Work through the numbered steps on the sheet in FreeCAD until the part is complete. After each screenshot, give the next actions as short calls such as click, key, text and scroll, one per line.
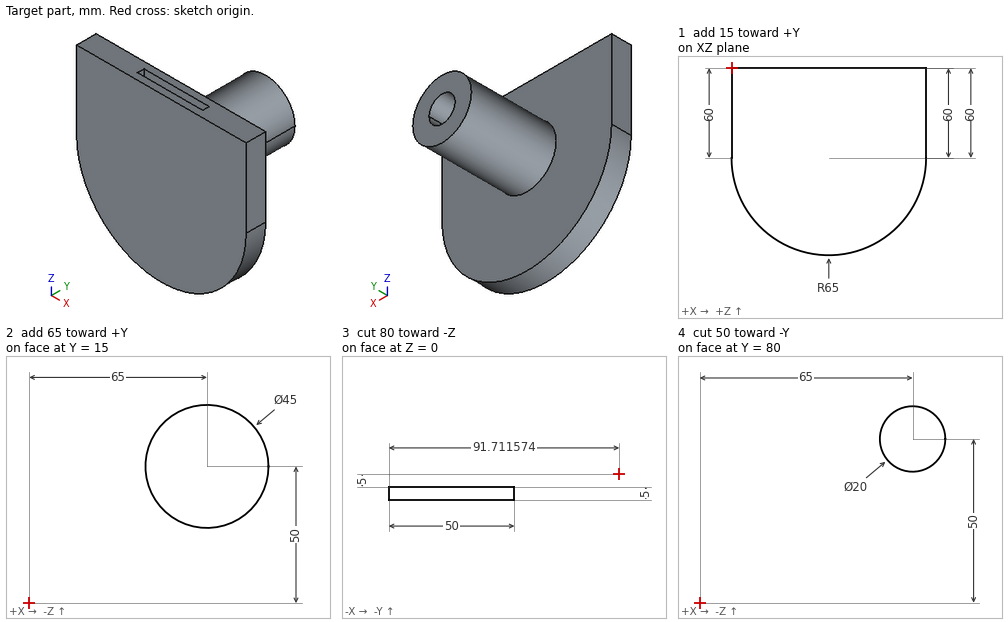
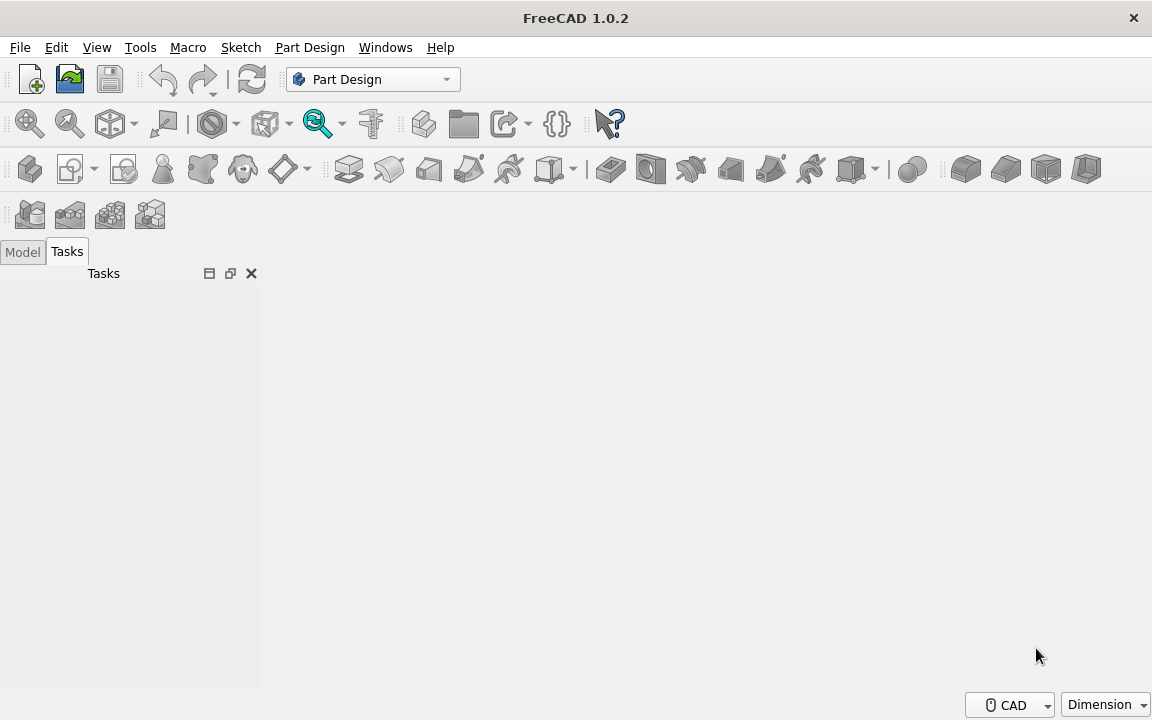
click(30, 170)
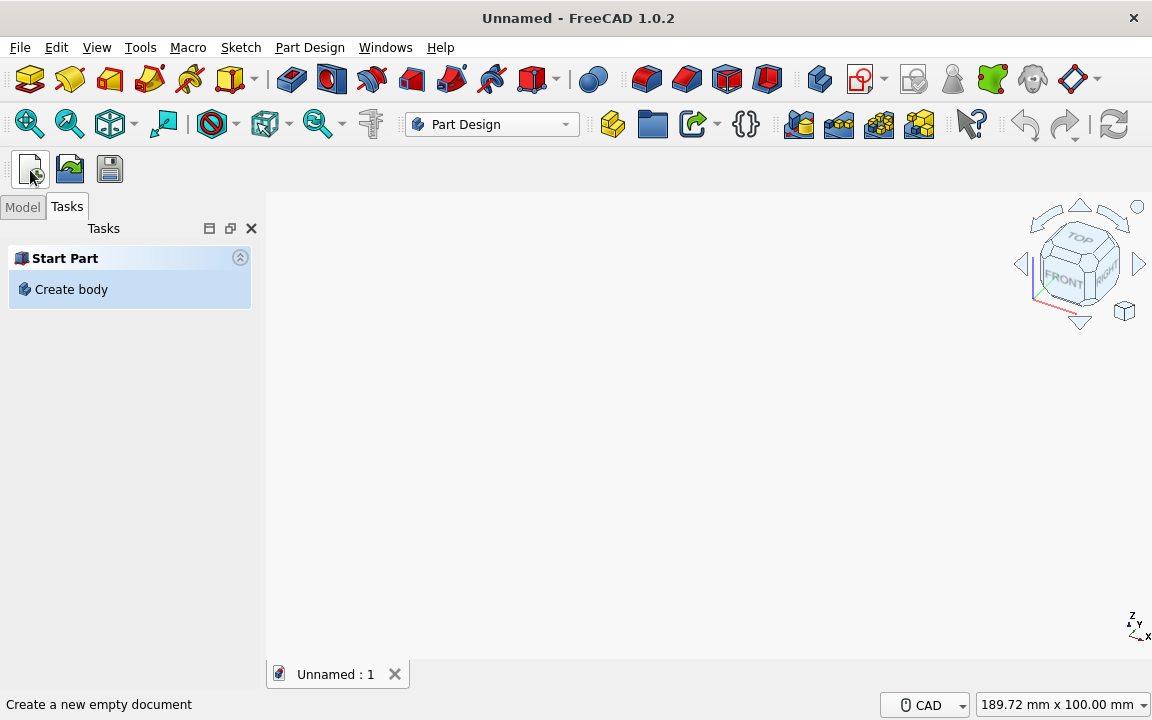
click(860, 80)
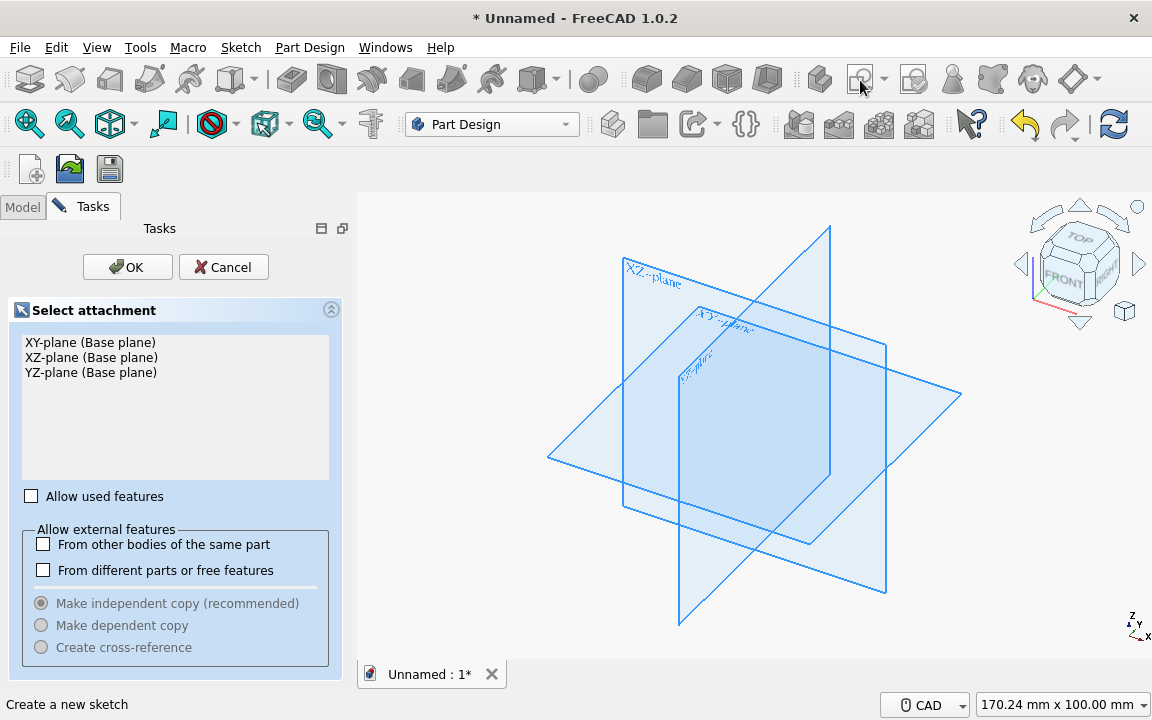
click(82, 358)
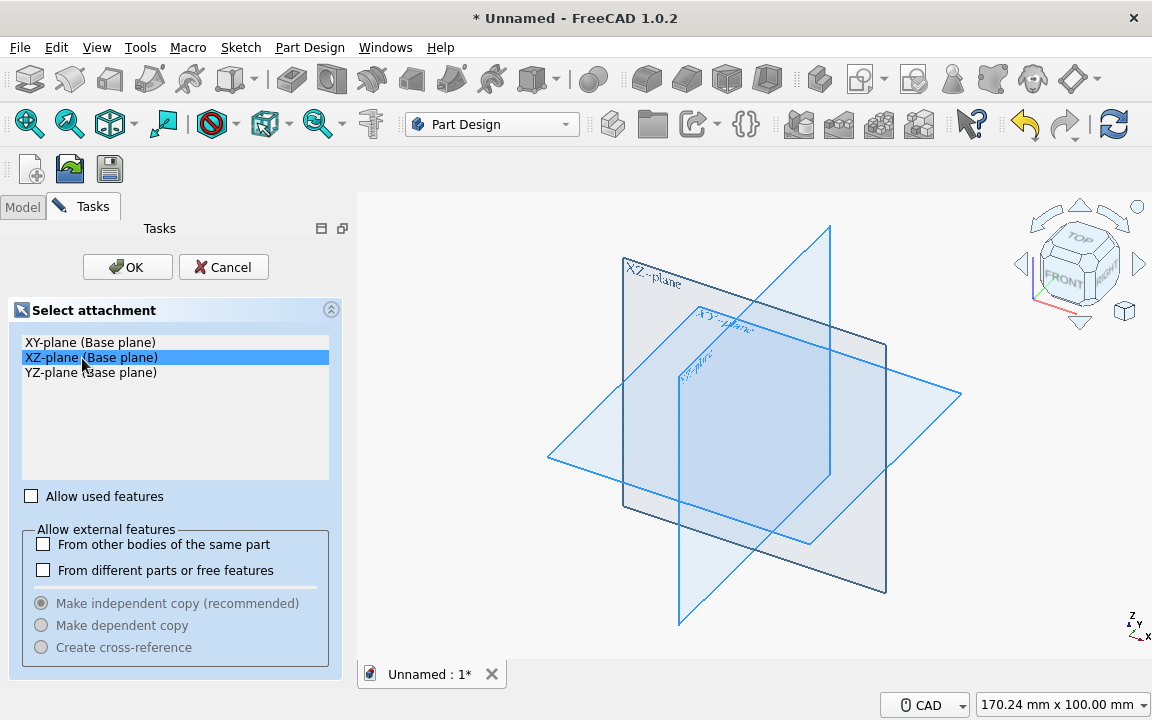
click(128, 267)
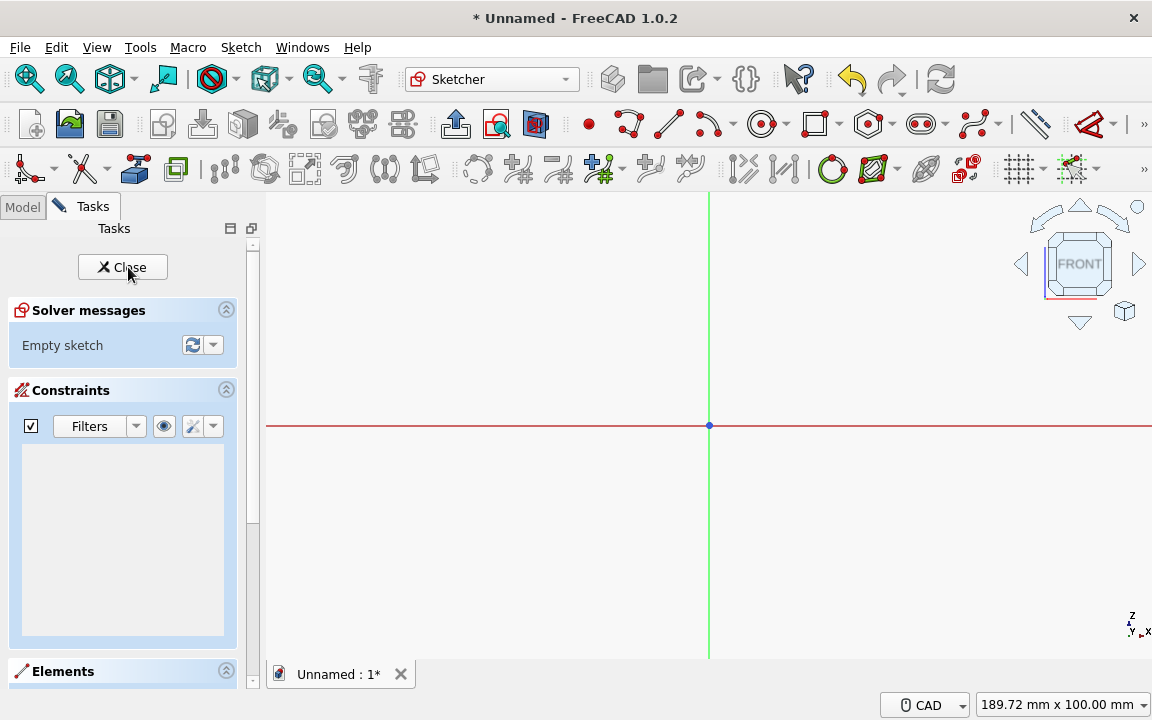
scroll(337, 220, down, 4)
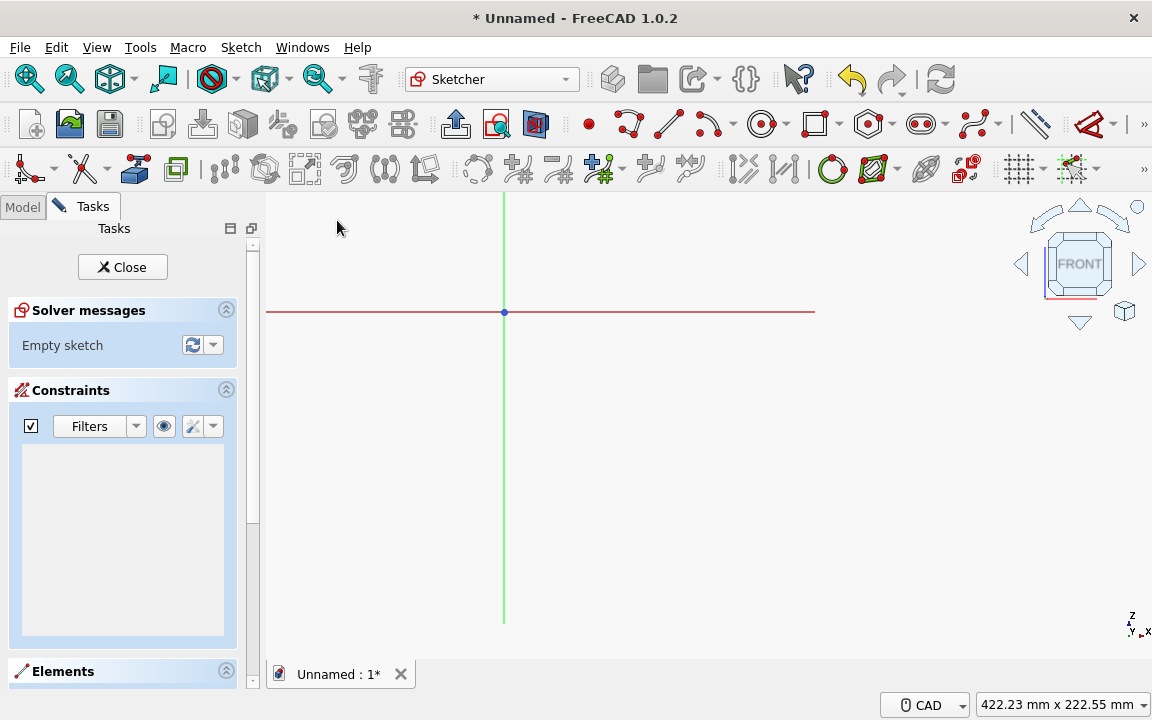
click(630, 124)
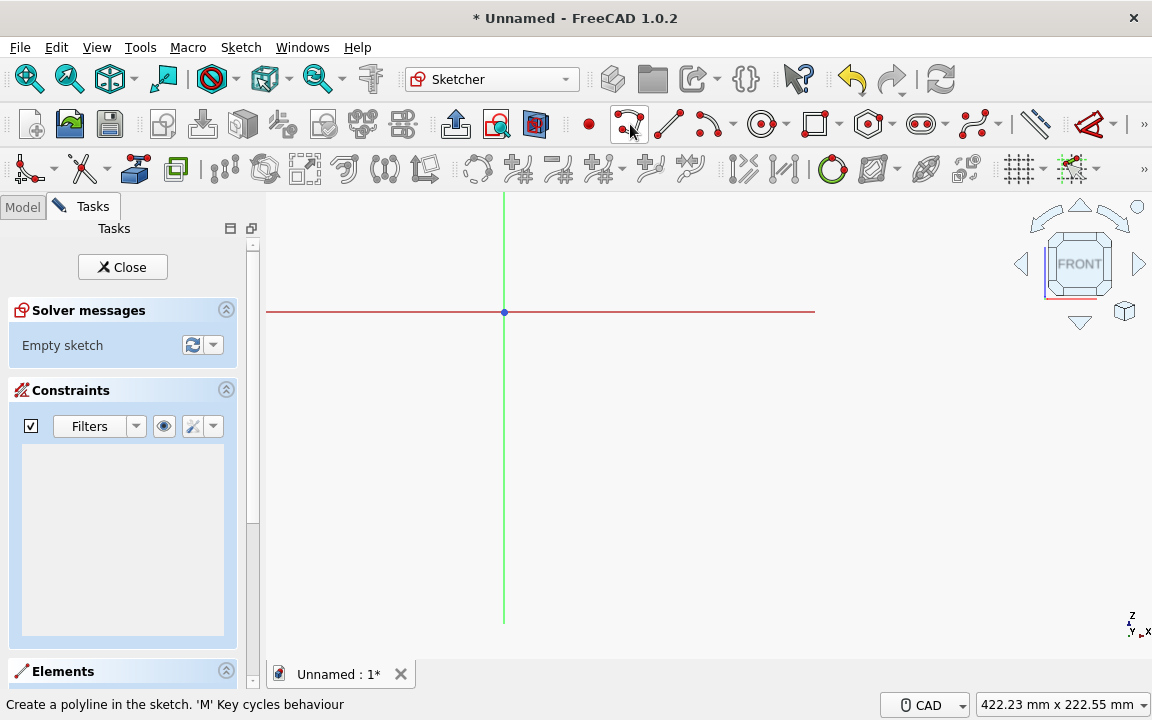
click(504, 438)
click(504, 312)
click(777, 321)
click(777, 438)
right_click(777, 438)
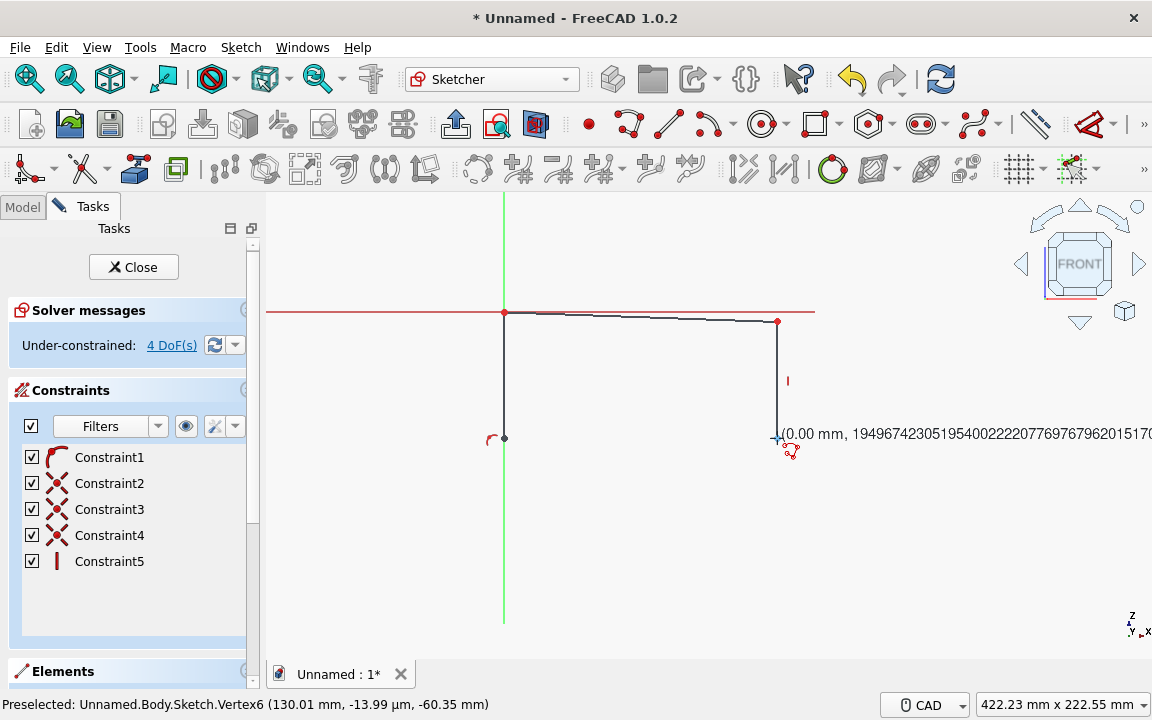
key(g)
key(3)
key(a)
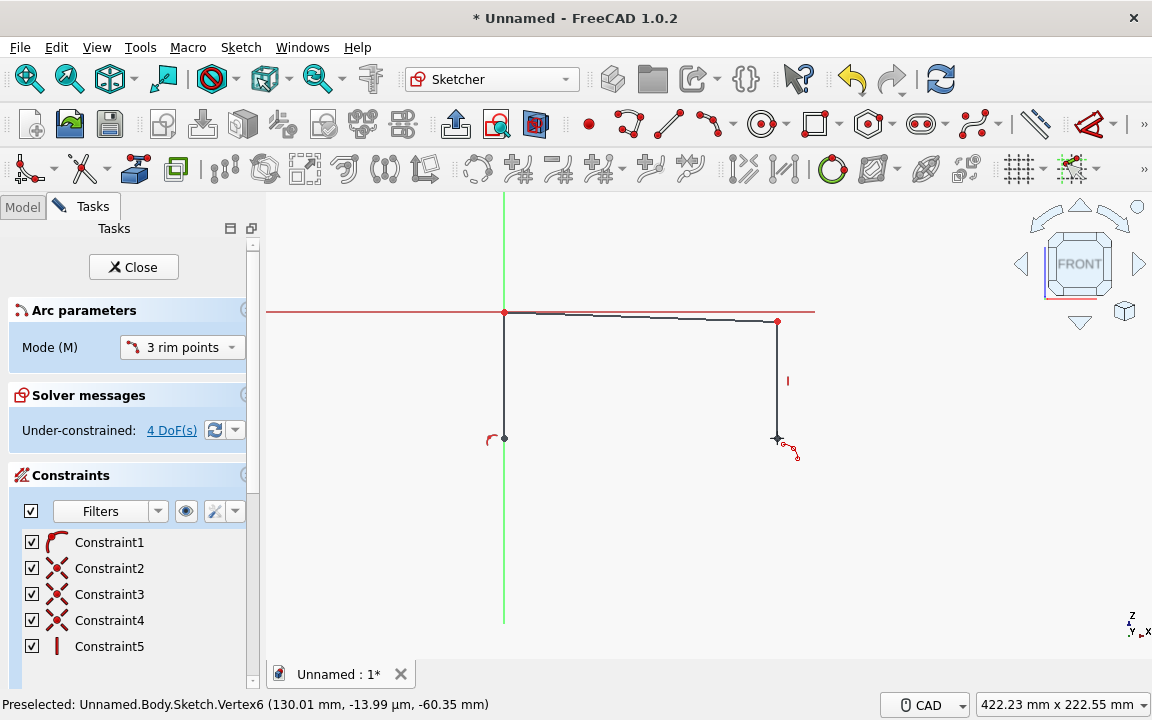
click(777, 439)
click(504, 439)
click(641, 575)
key(Escape)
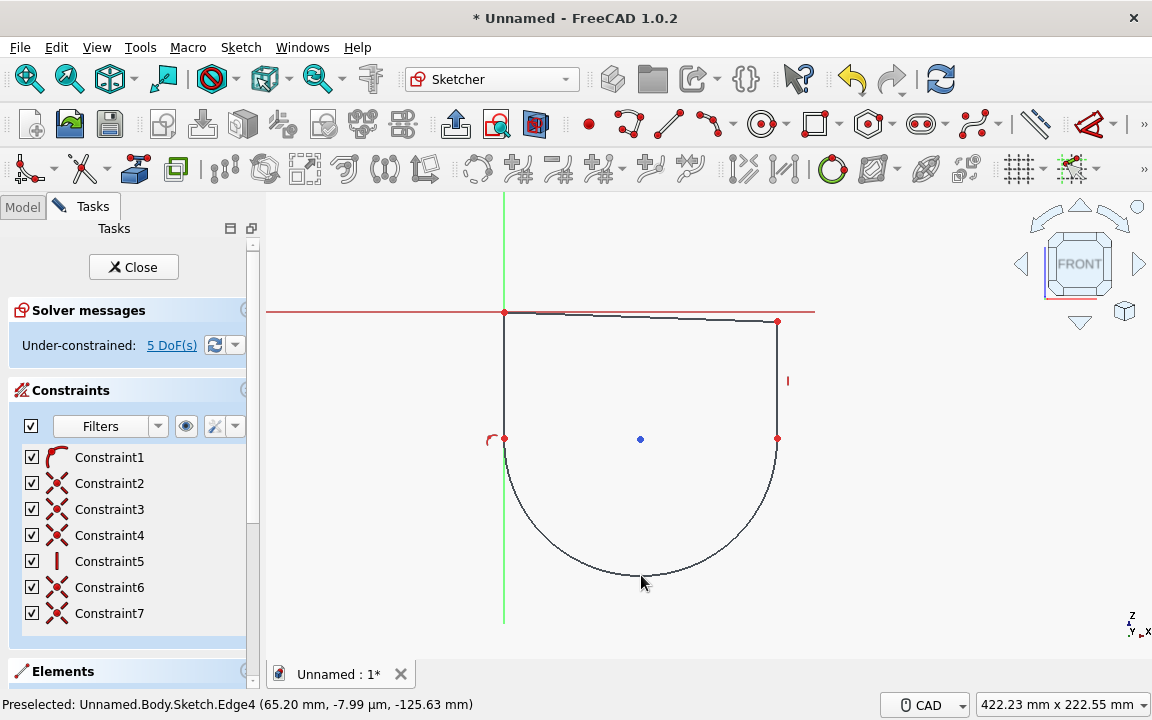
click(586, 315)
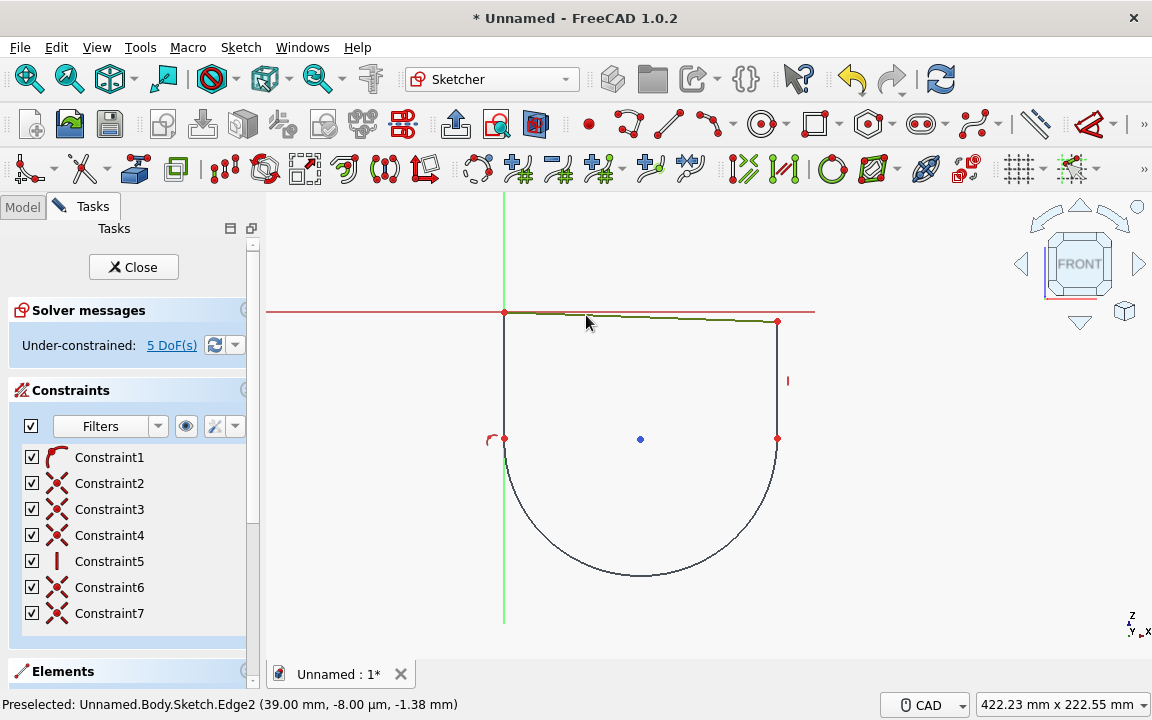
key(h)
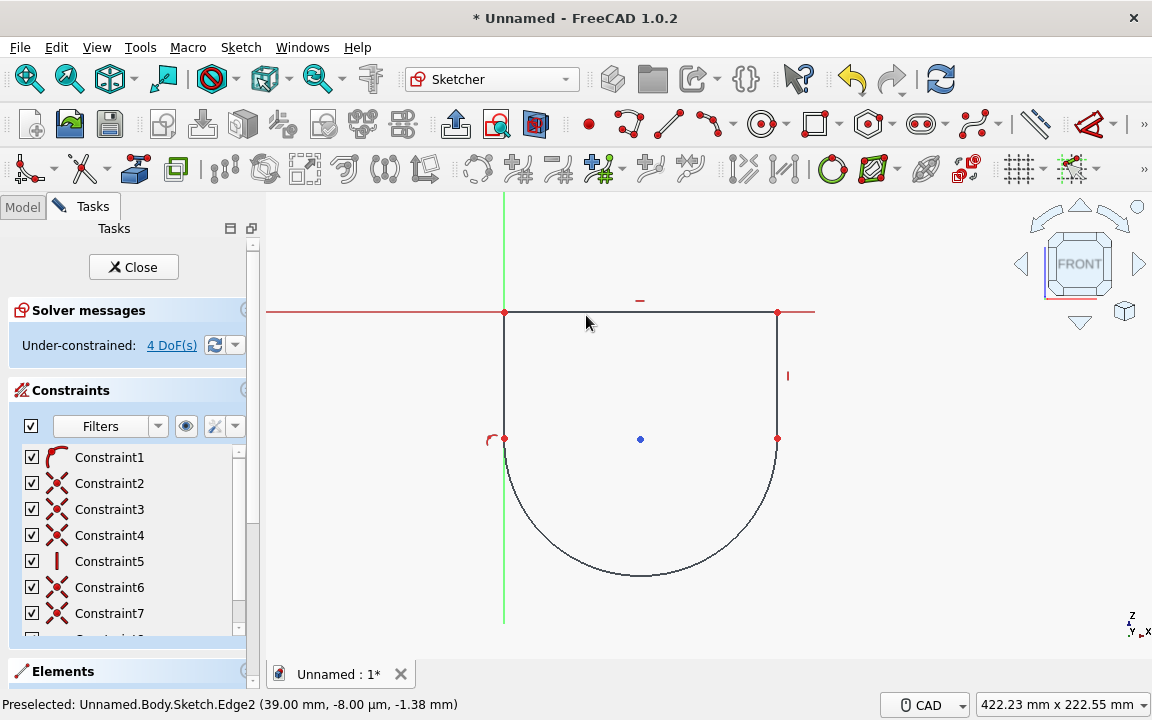
click(560, 550)